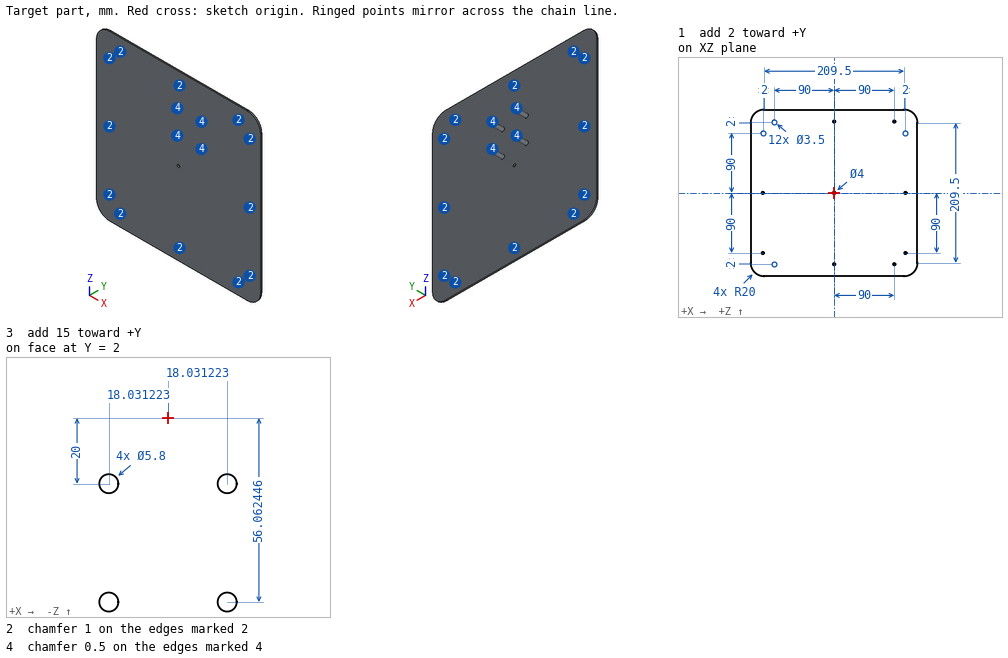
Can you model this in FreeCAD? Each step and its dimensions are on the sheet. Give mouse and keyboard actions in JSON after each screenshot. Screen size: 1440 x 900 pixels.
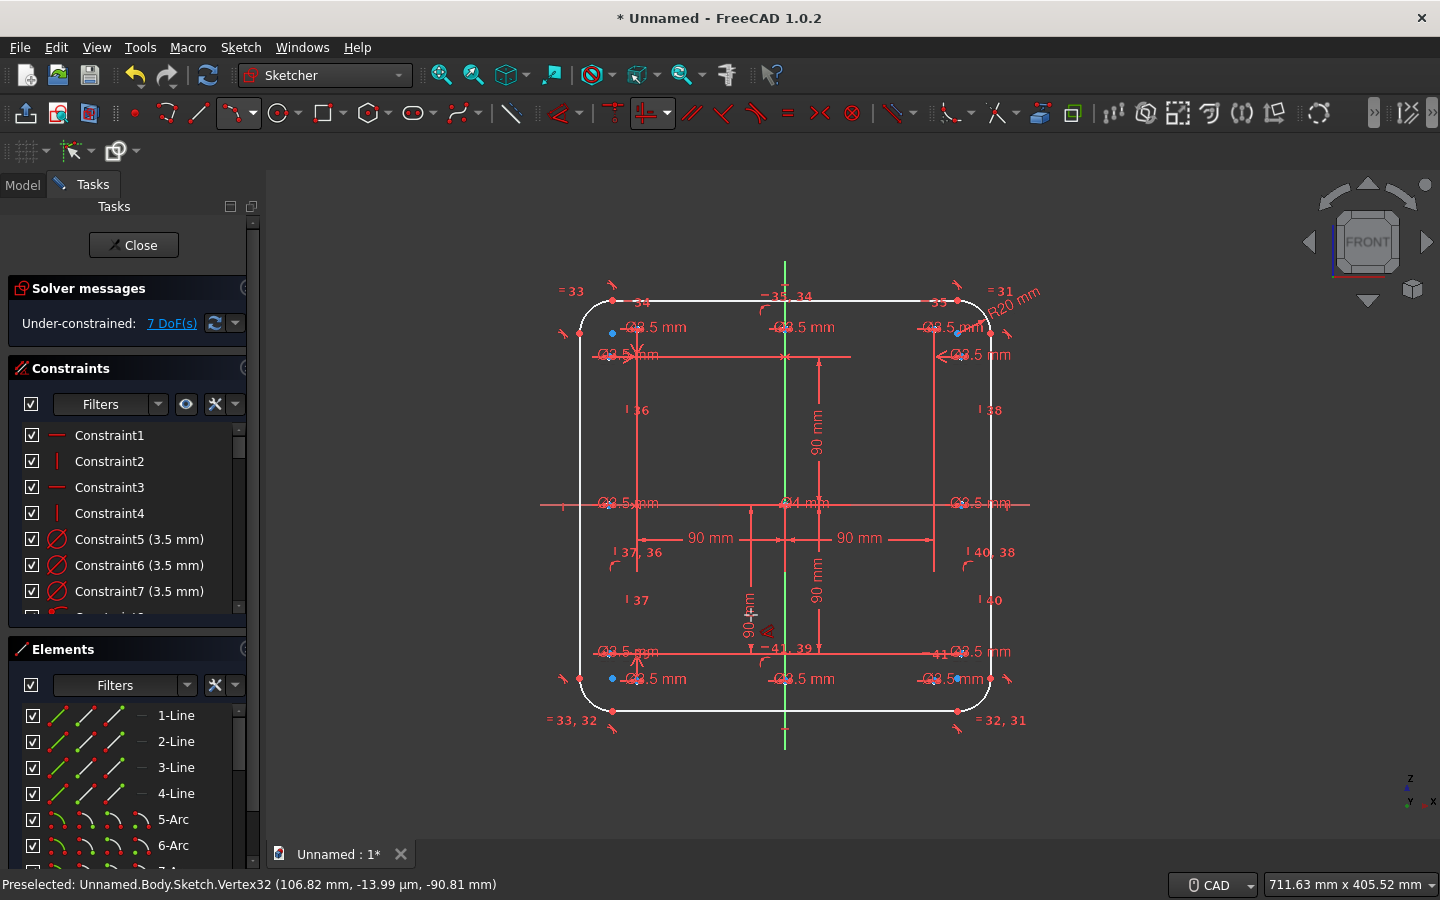
{"action": "left_click", "coordinate": [934, 681]}
{"action": "left_click", "coordinate": [860, 471]}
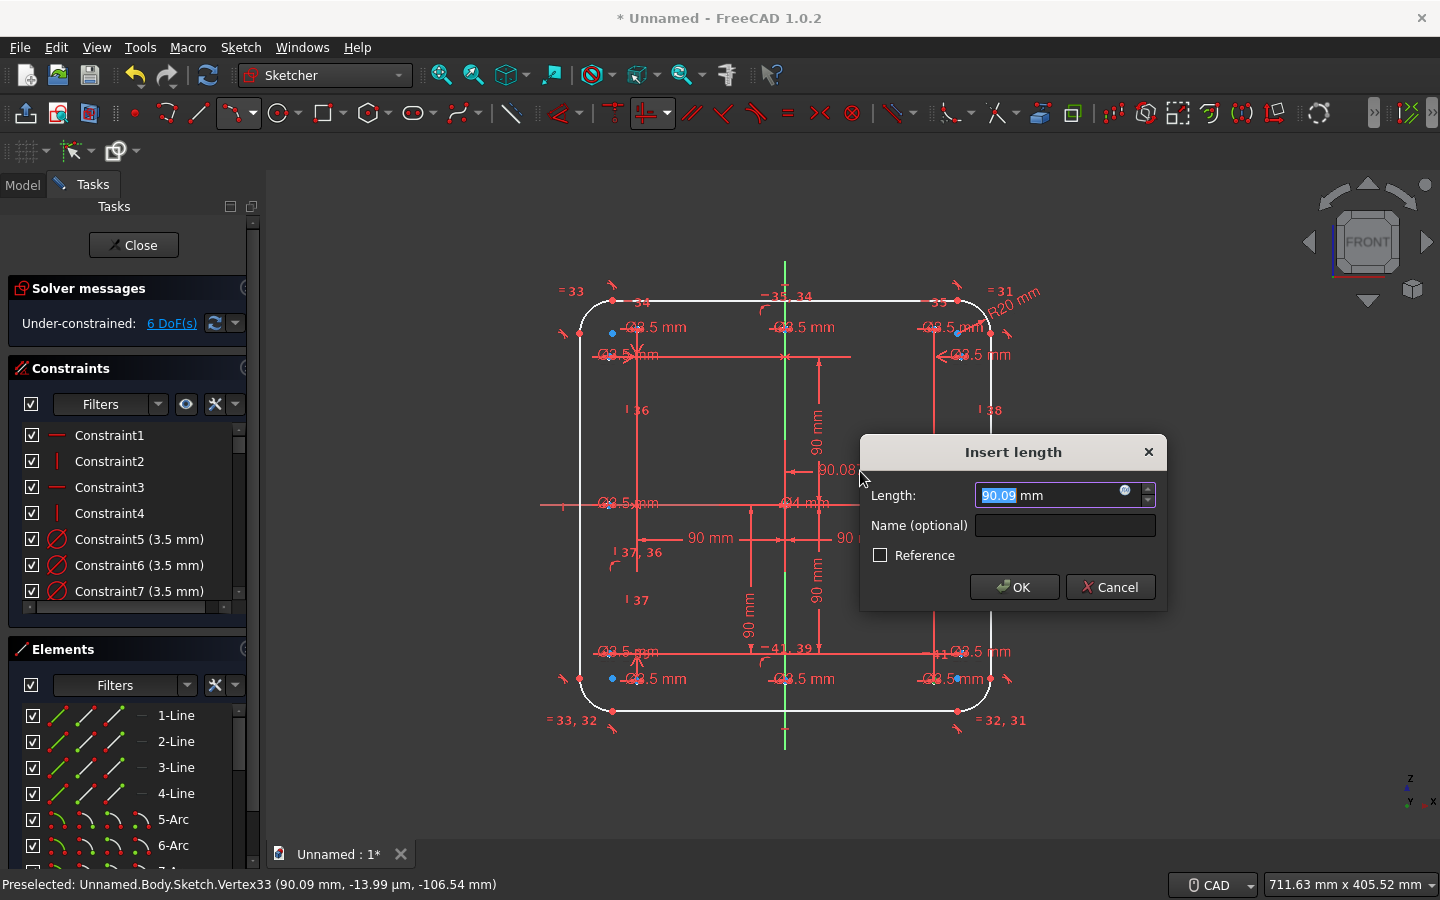
{"action": "type", "text": "90"}
{"action": "key", "text": "Return"}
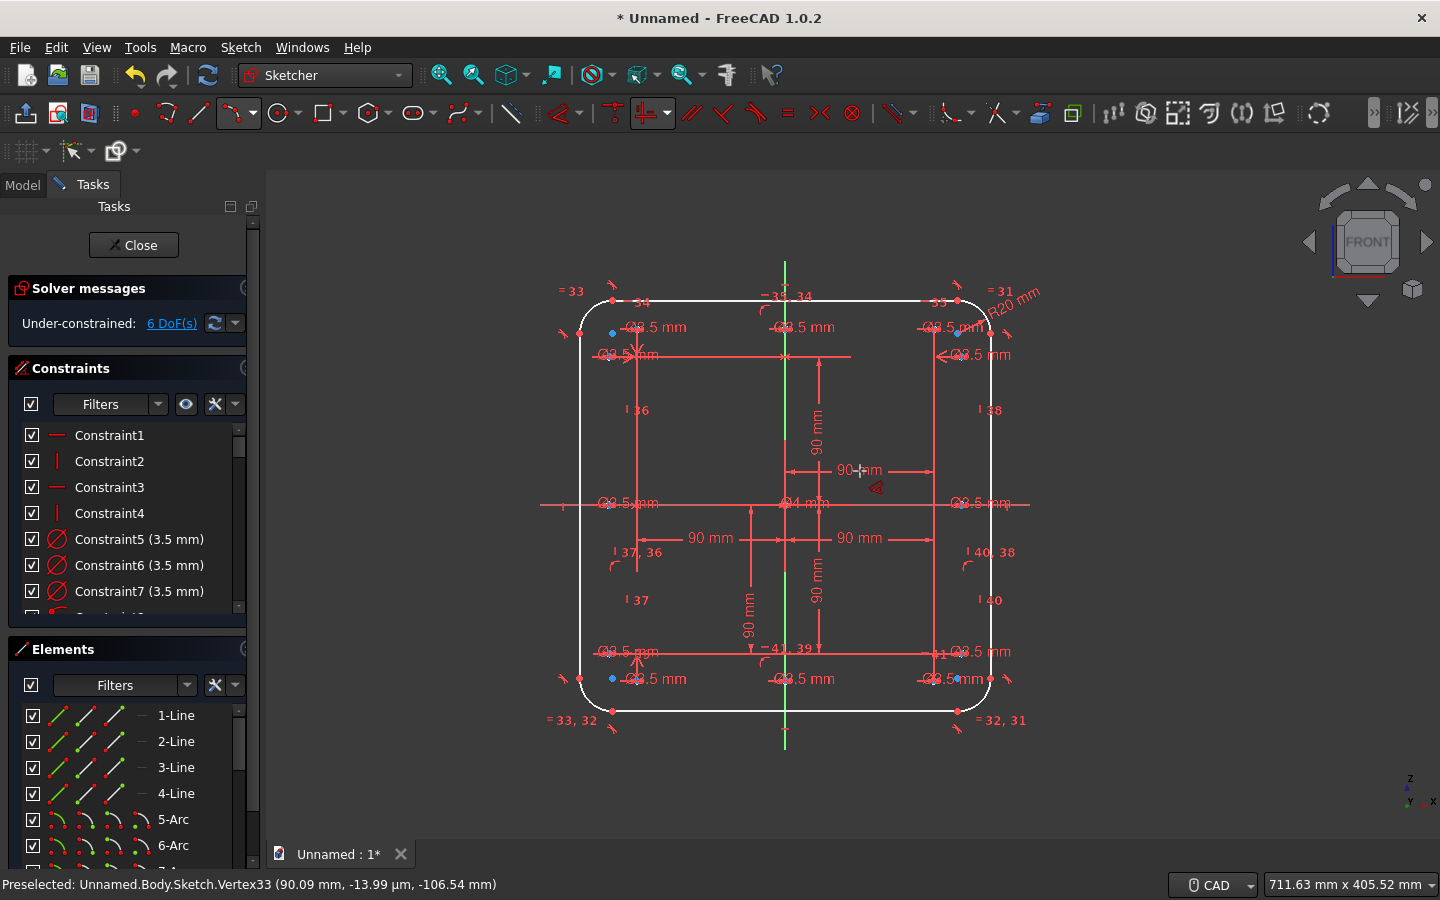
{"action": "scroll", "coordinate": [580, 334], "scroll_direction": "up", "scroll_amount": 13}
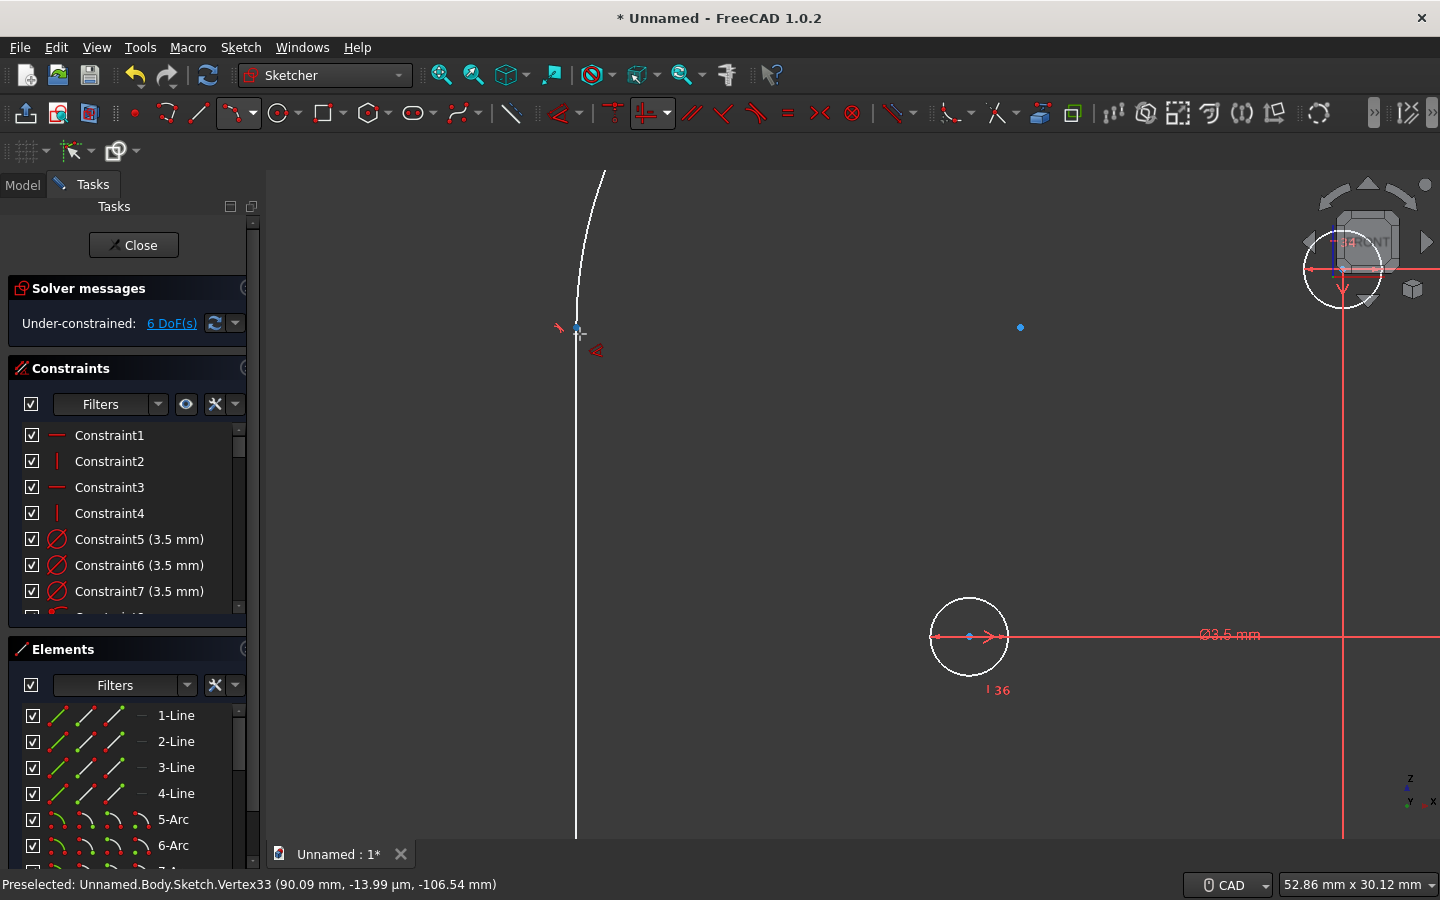
{"action": "left_click", "coordinate": [576, 328]}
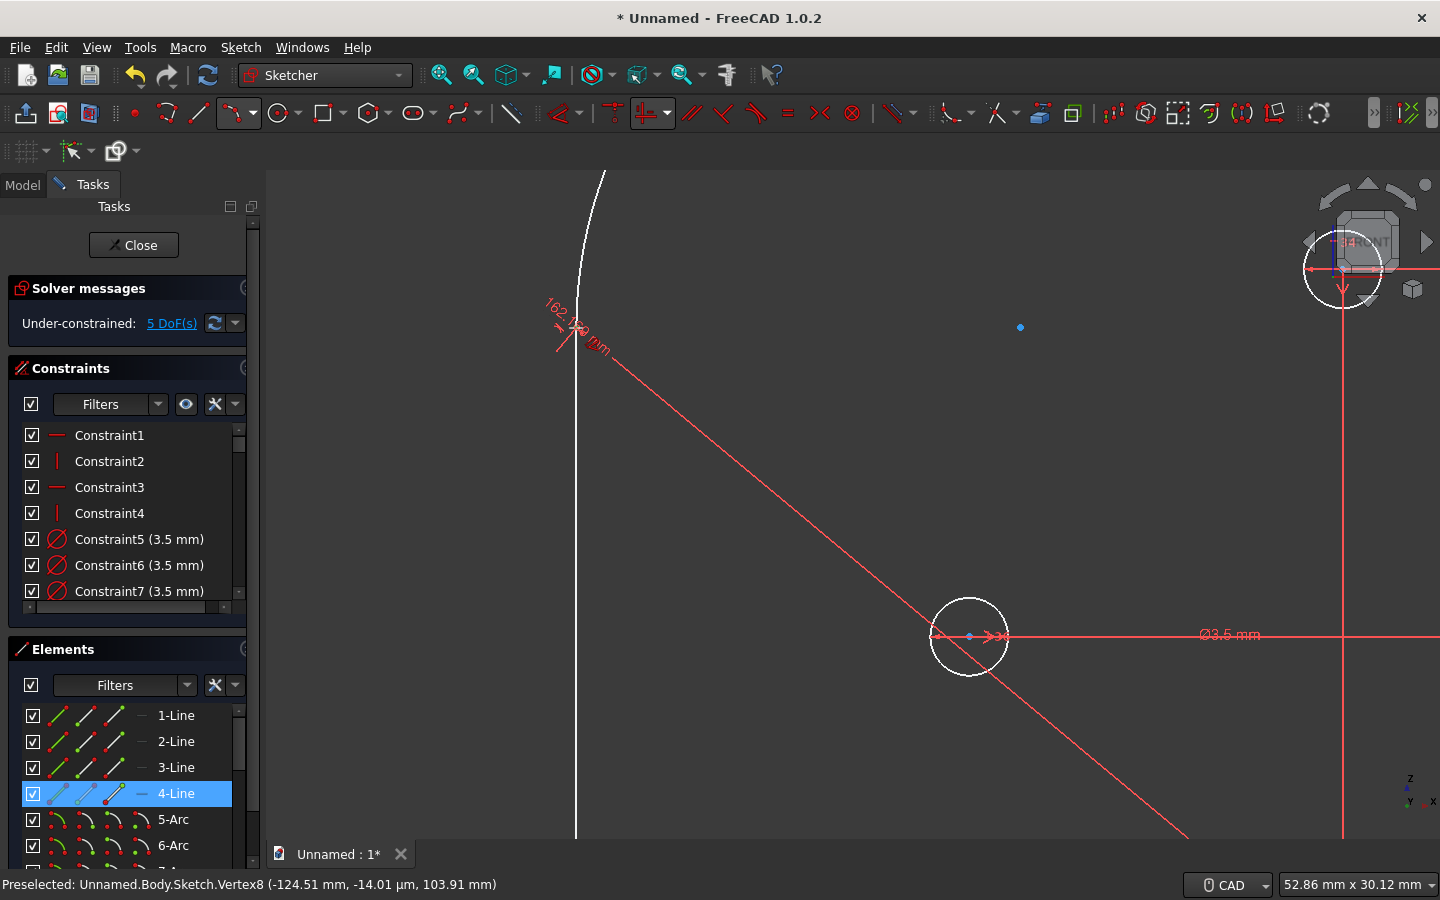
{"action": "scroll", "coordinate": [579, 334], "scroll_direction": "down", "scroll_amount": 13}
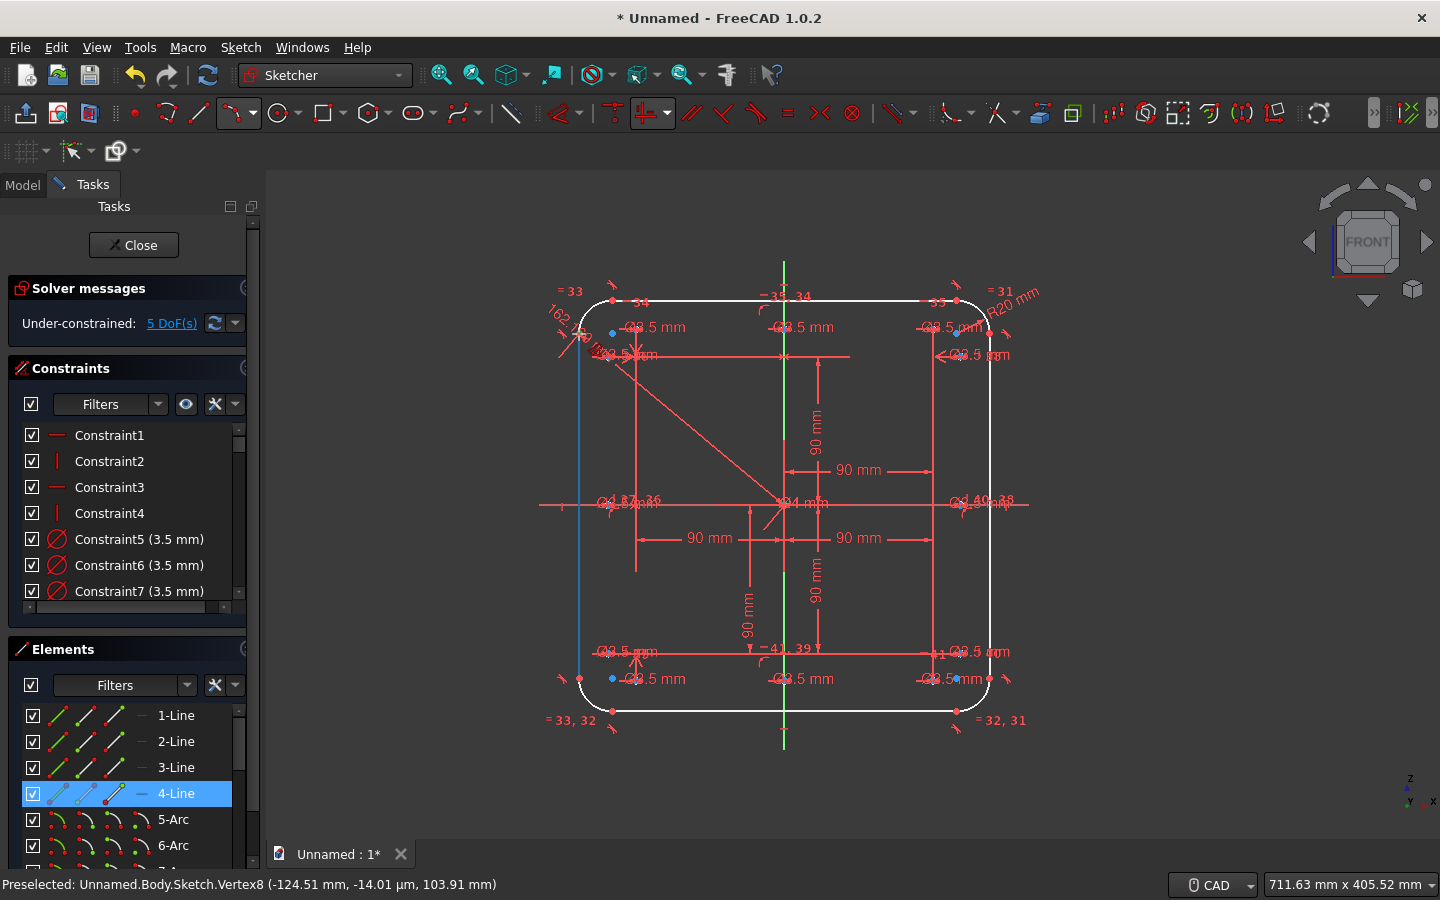
{"action": "scroll", "coordinate": [636, 329], "scroll_direction": "up", "scroll_amount": 13}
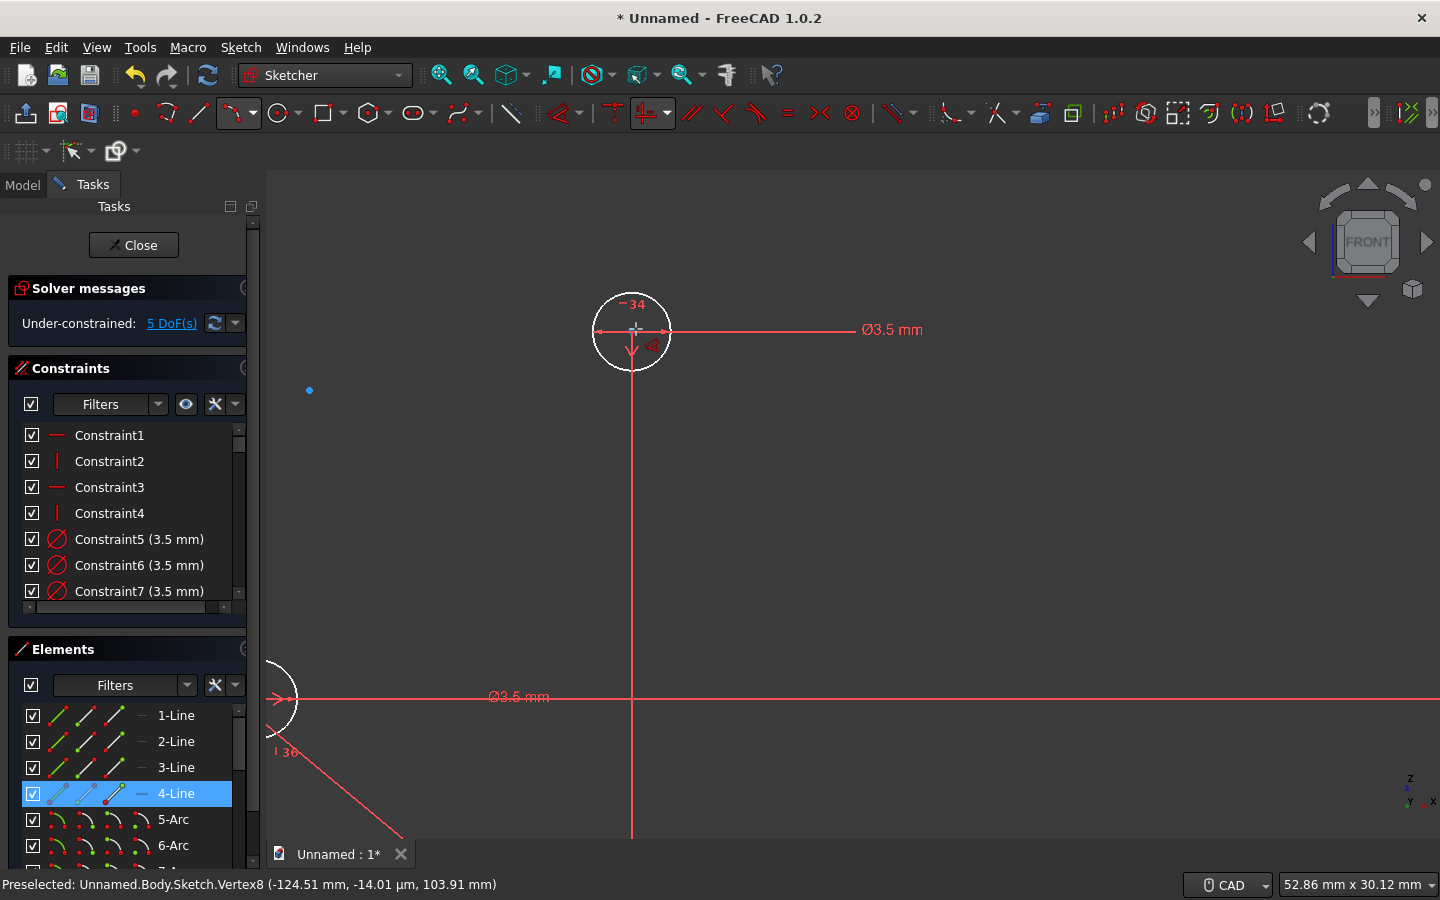
{"action": "left_click", "coordinate": [632, 332]}
{"action": "left_click", "coordinate": [666, 374]}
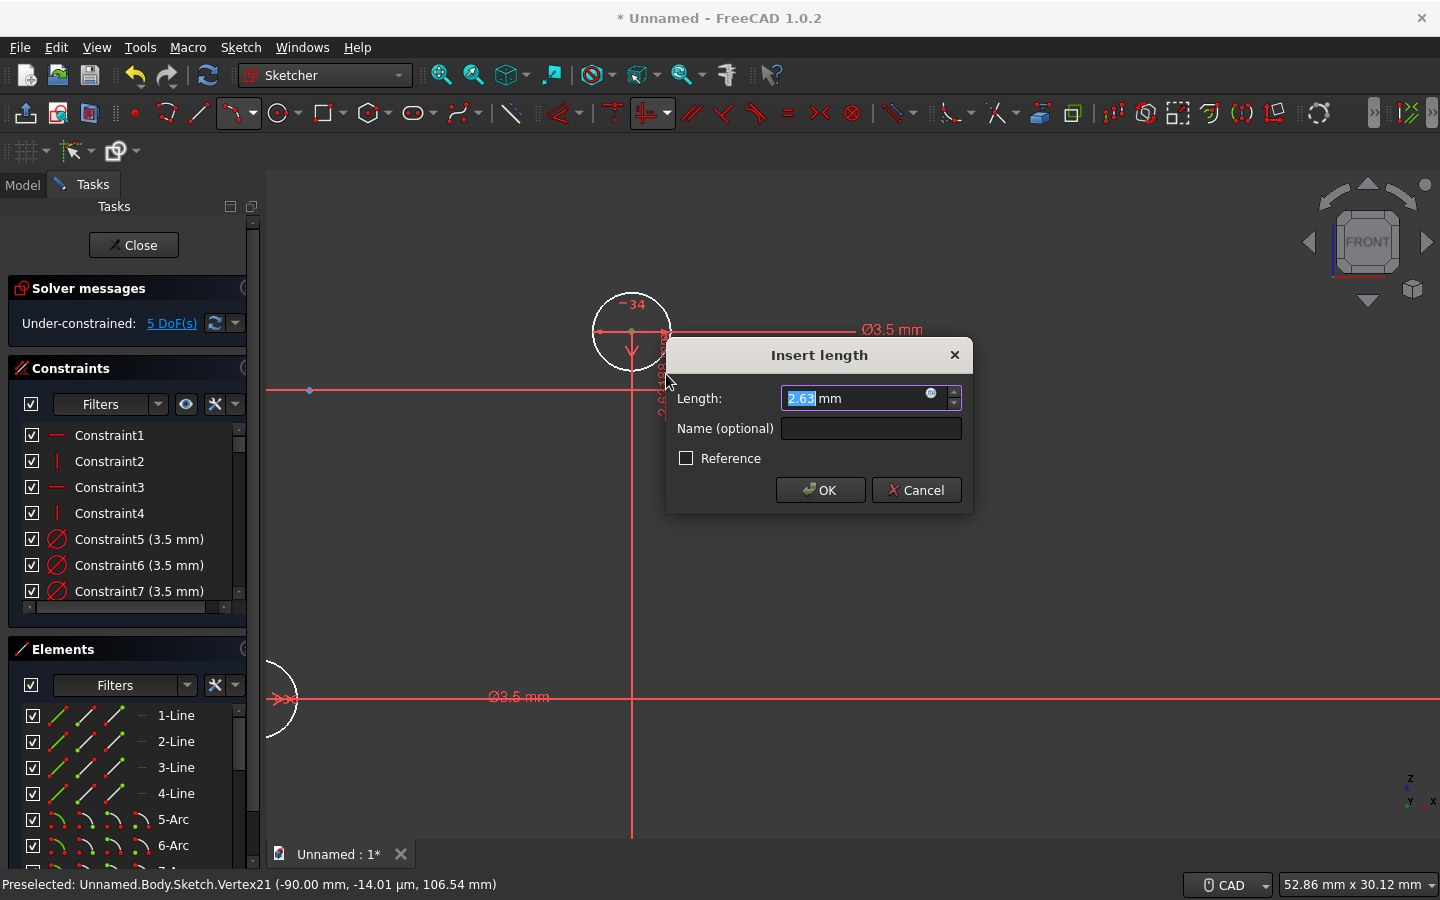
{"action": "type", "text": "2"}
{"action": "key", "text": "Return"}